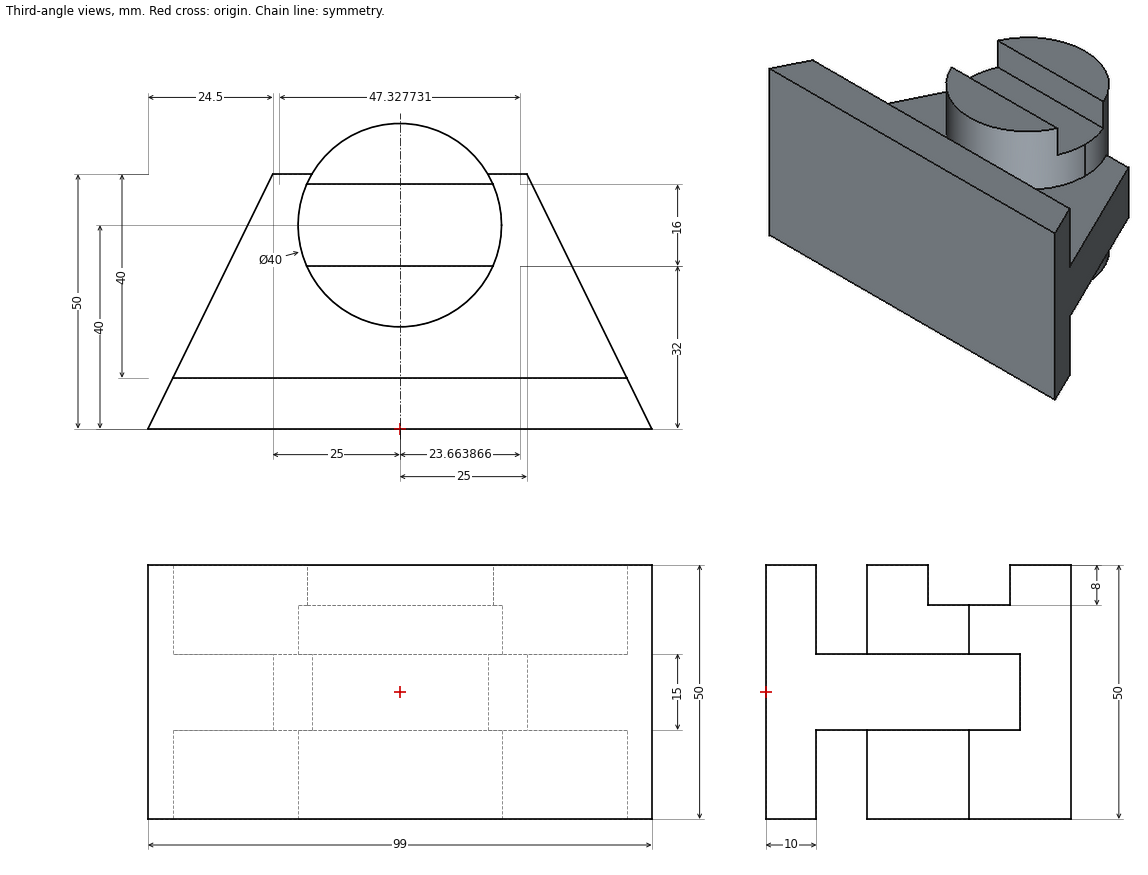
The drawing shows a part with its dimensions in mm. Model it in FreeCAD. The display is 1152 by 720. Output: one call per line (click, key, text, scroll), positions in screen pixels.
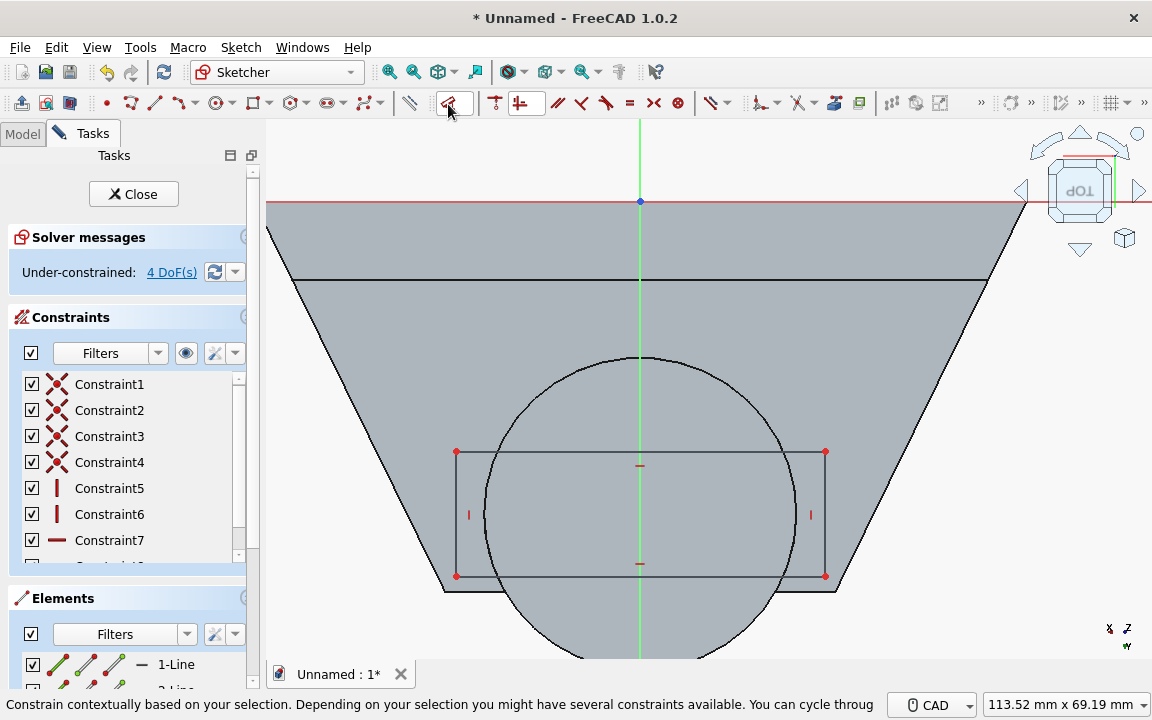
click(456, 490)
click(422, 514)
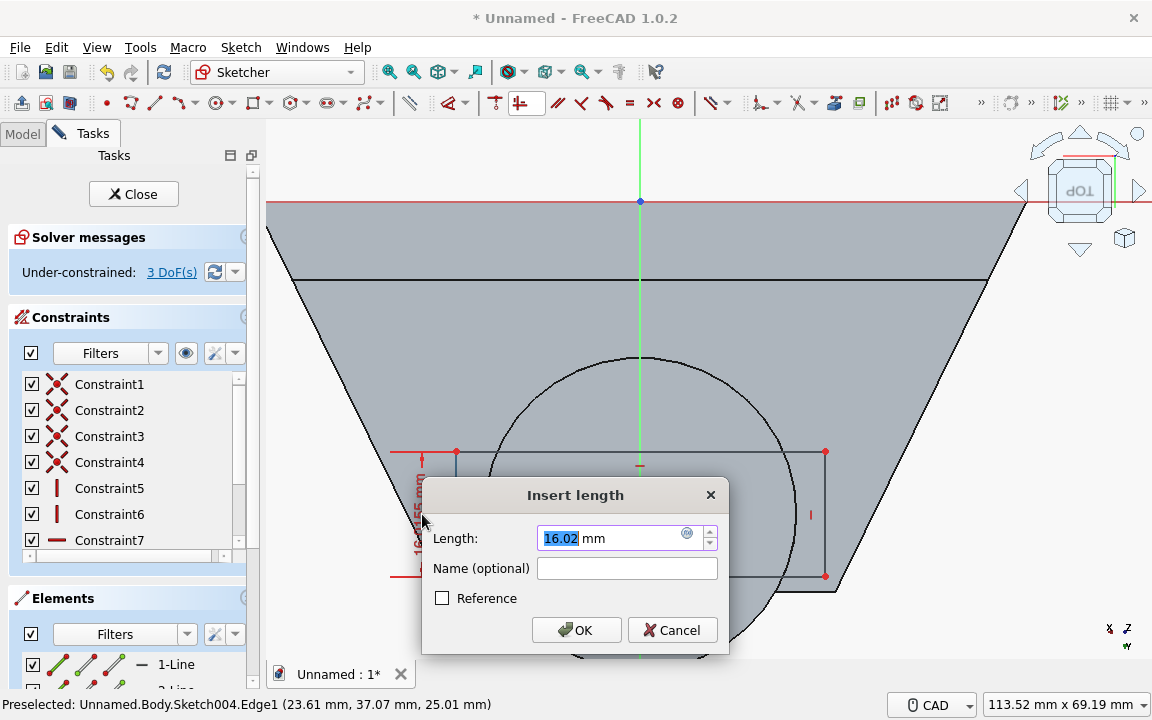
text(16)
key(Return)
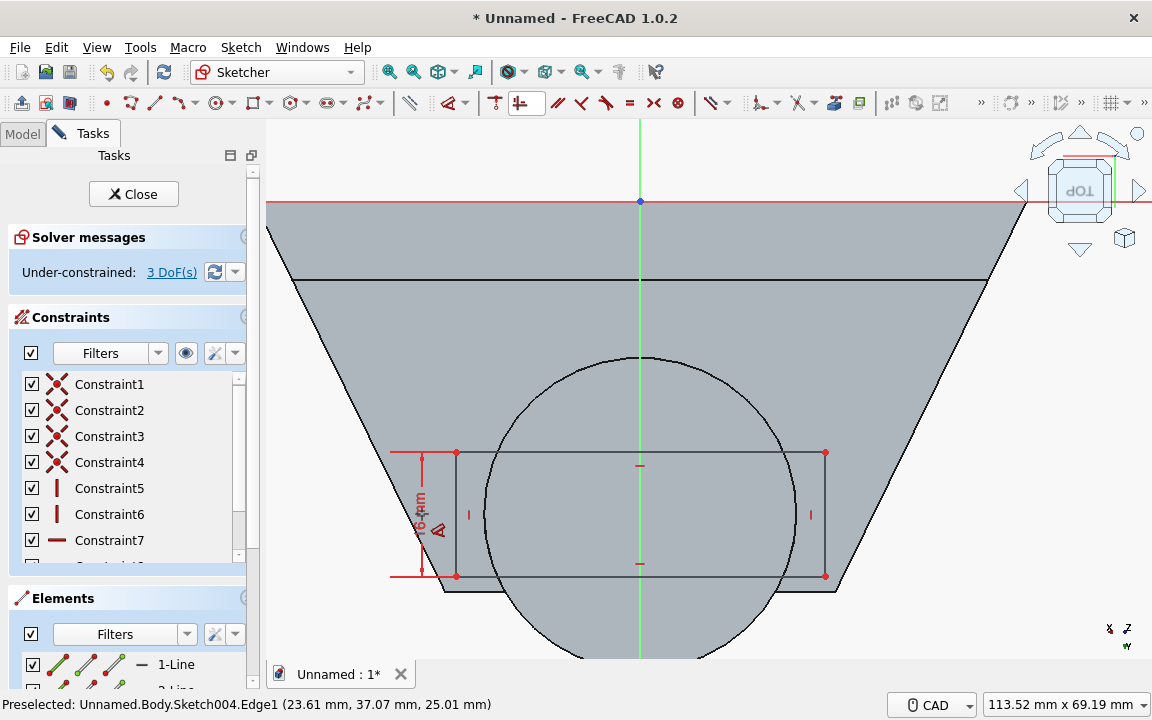
click(456, 452)
click(422, 327)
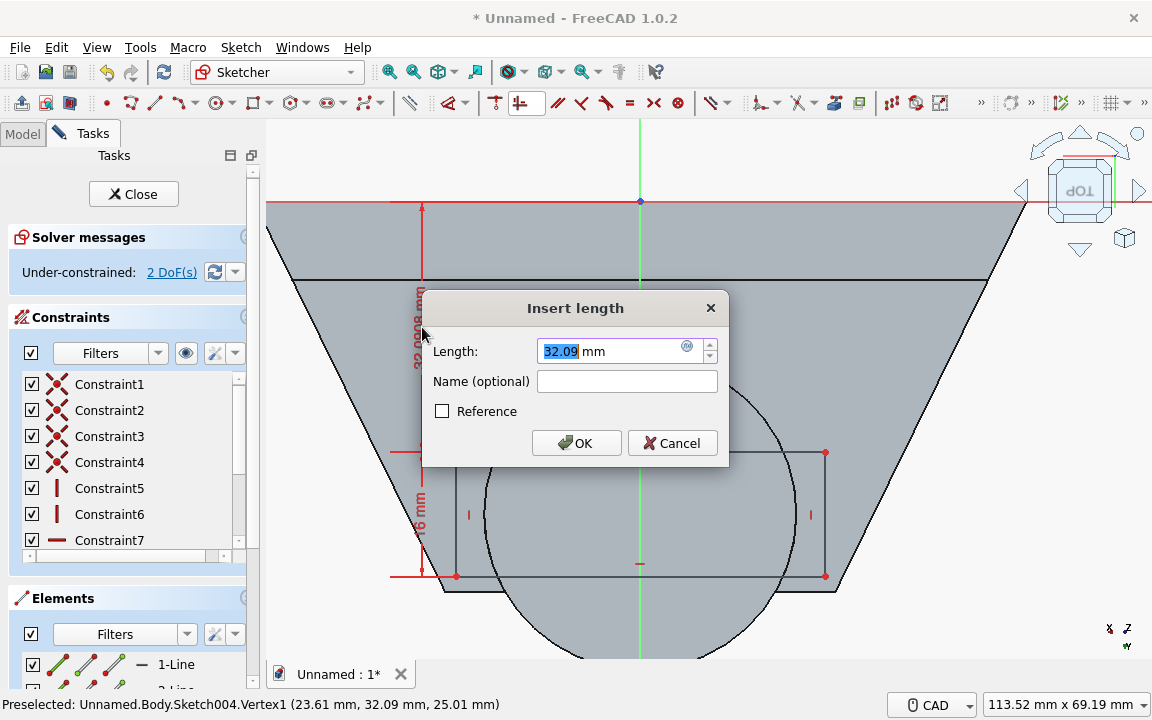
text(32)
key(Return)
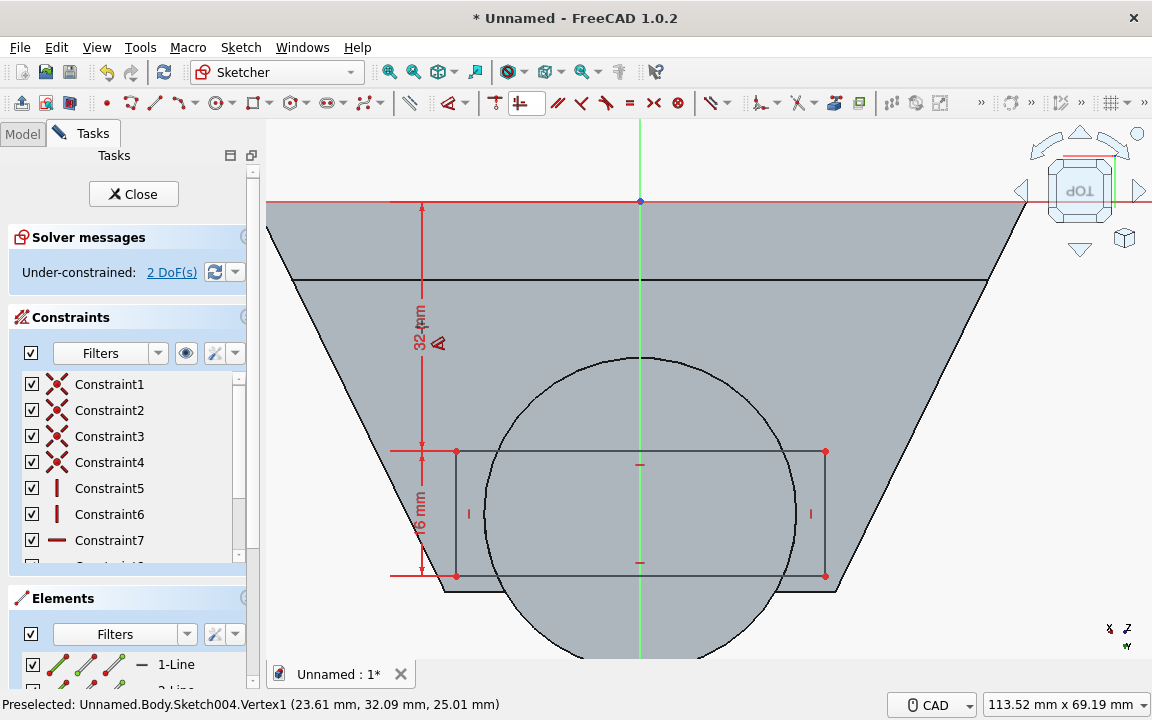
click(567, 576)
click(556, 610)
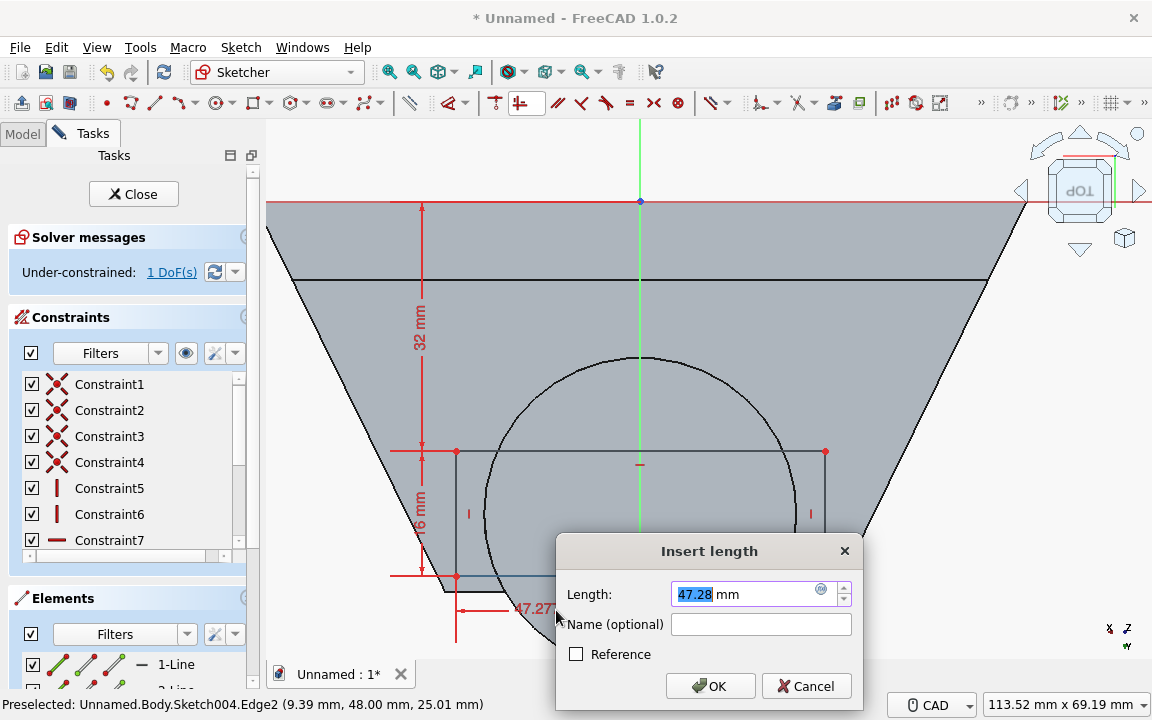
text(47.327731)
key(Return)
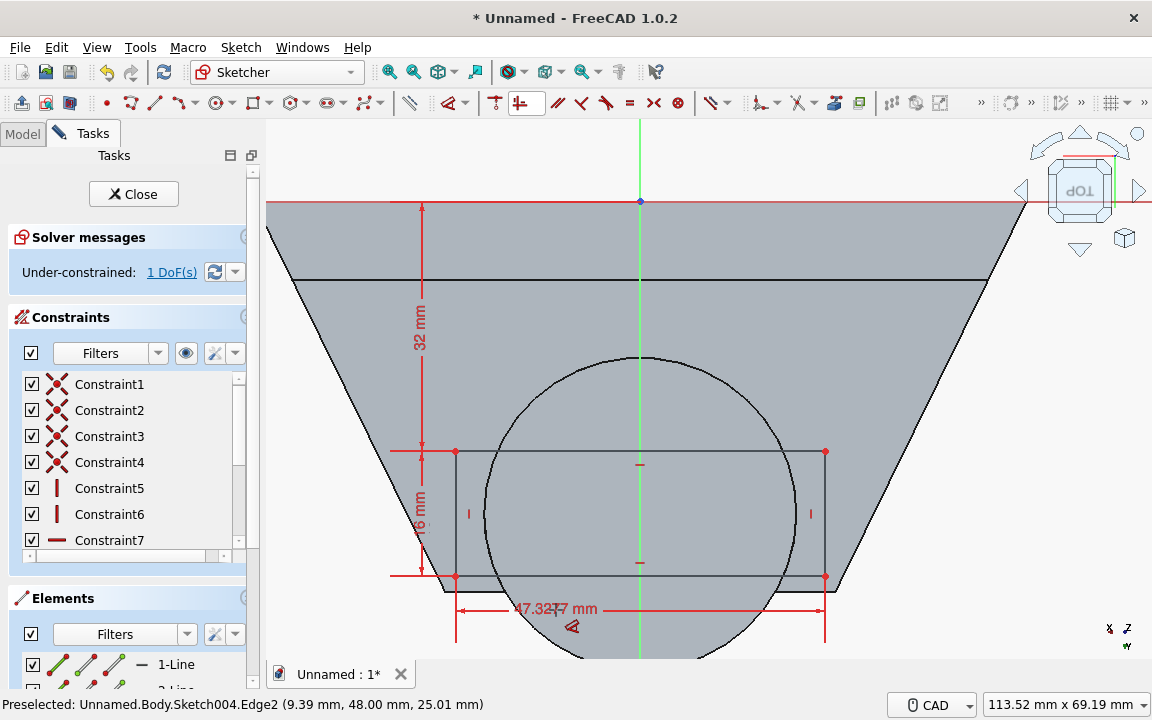
click(456, 451)
click(548, 168)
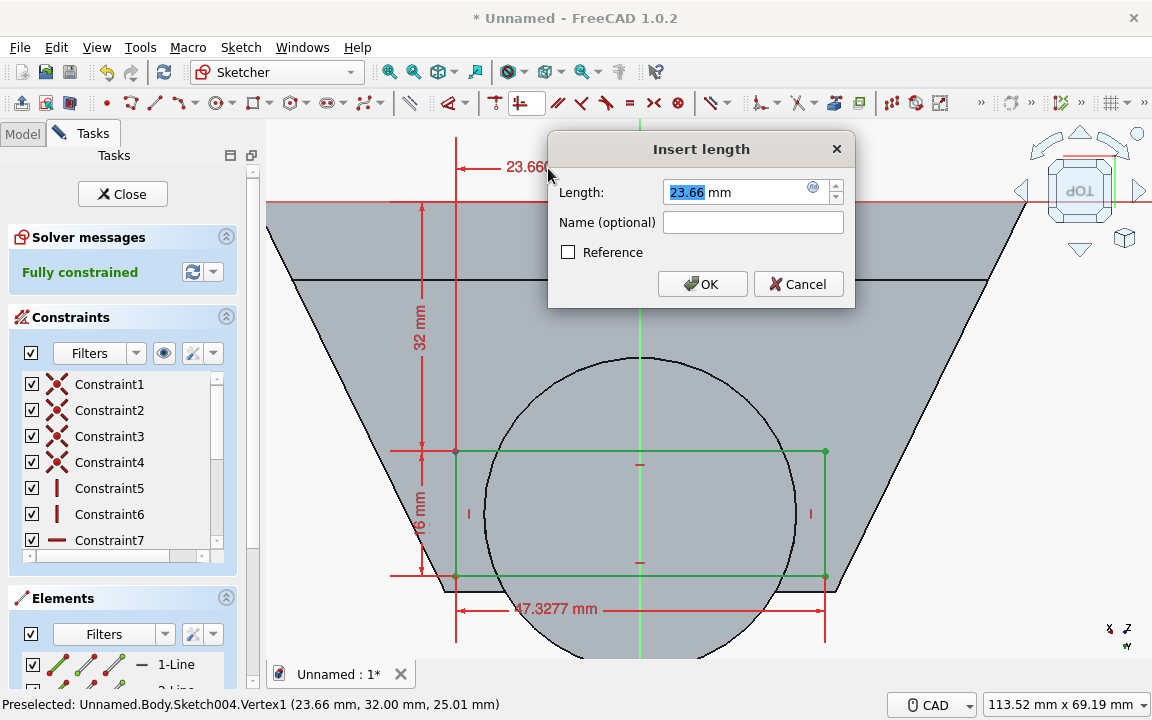
text(23.663866)
key(Return)
key(Escape)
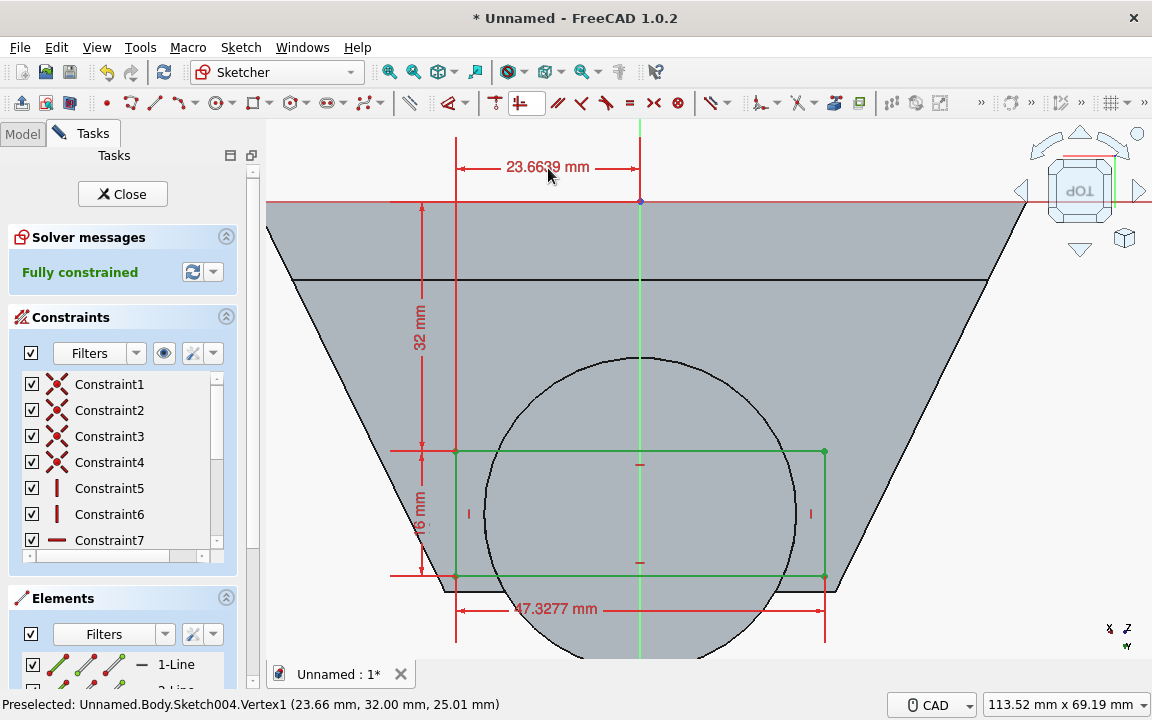
click(123, 194)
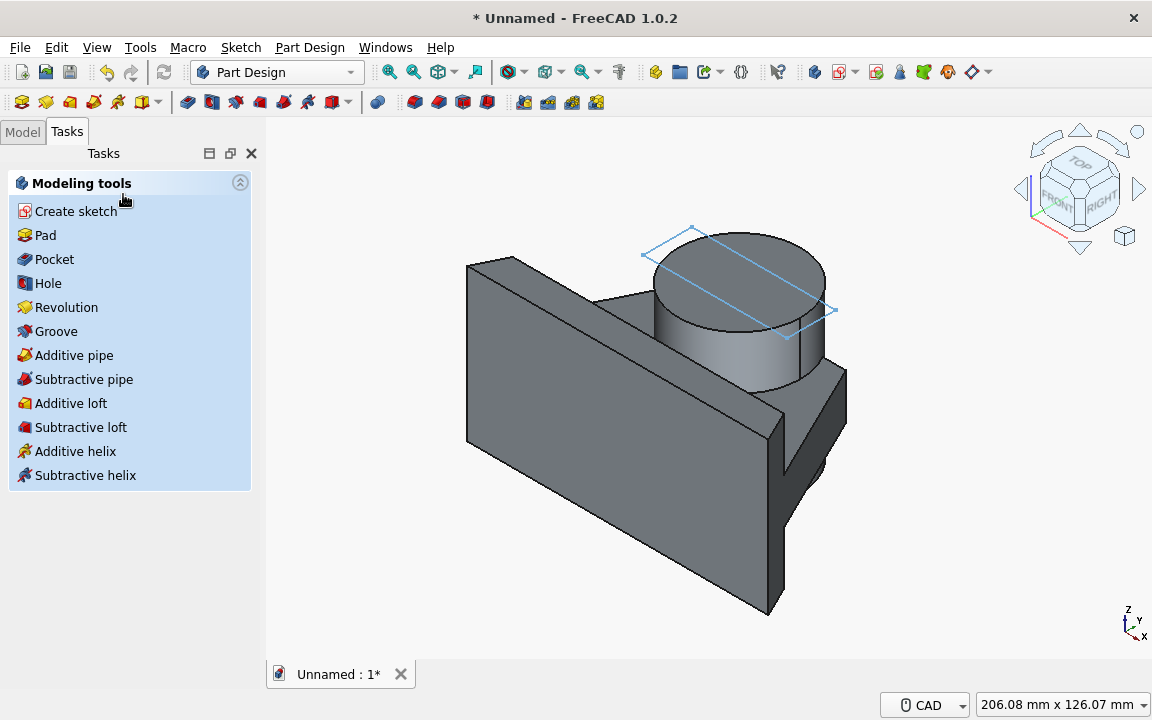
click(188, 102)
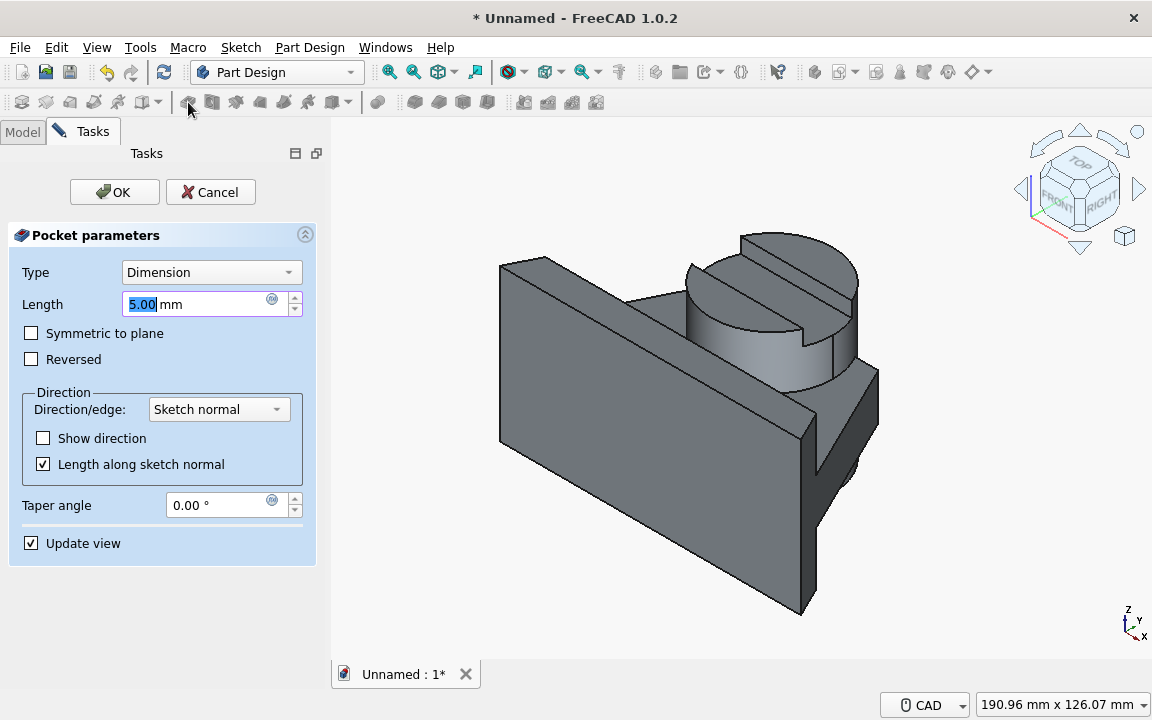
text(8)
key(Tab)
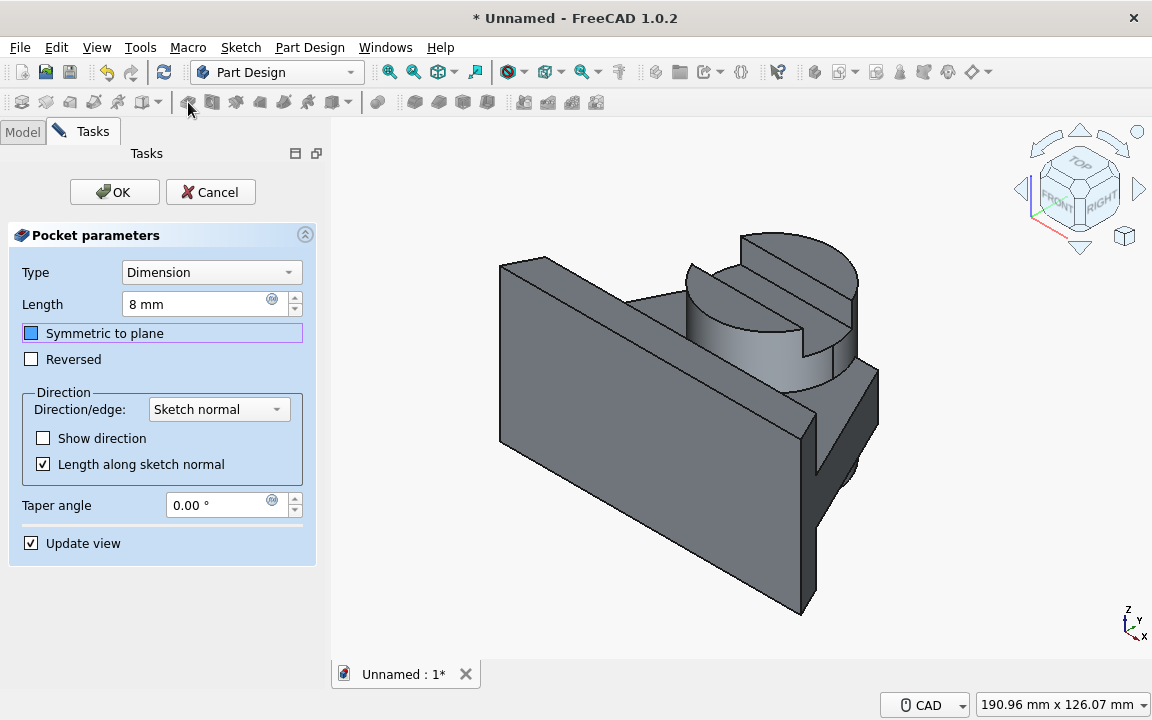
click(115, 192)